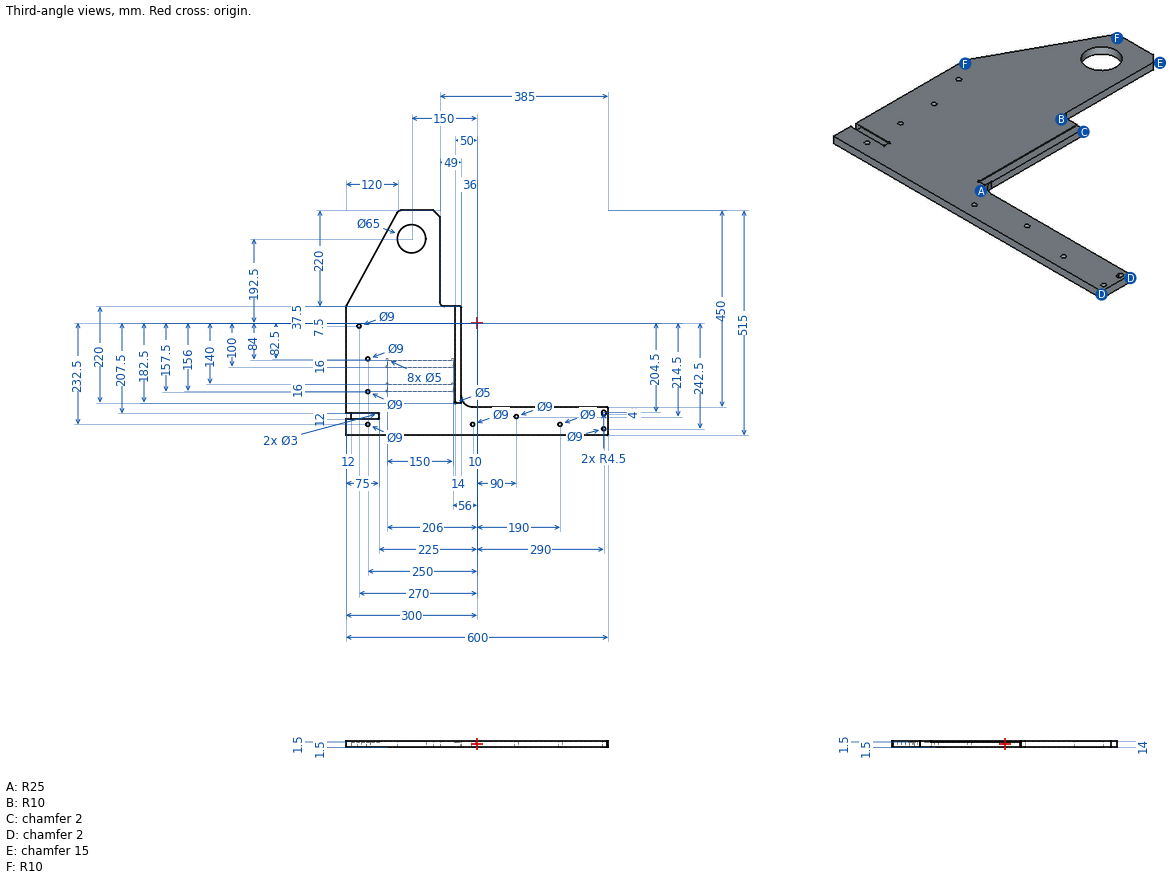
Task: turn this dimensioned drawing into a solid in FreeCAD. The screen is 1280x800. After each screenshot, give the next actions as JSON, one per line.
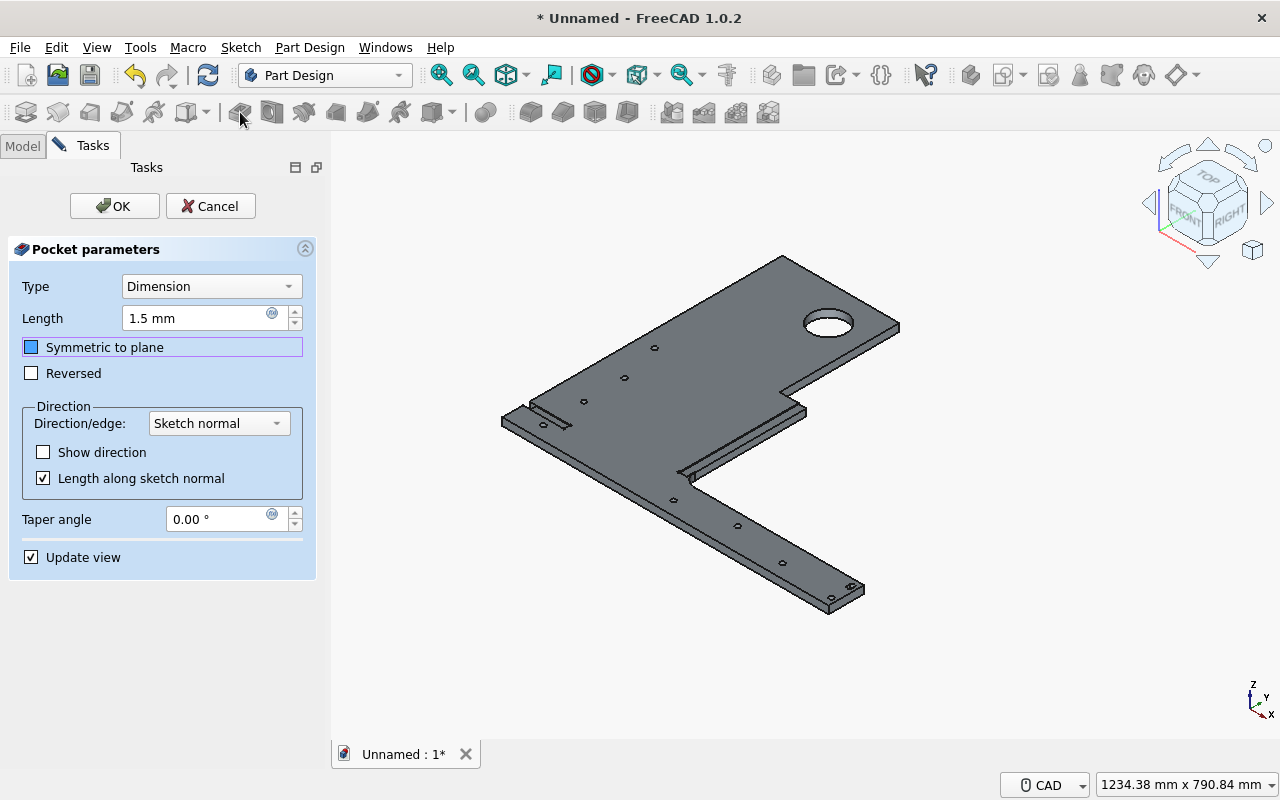
{"action": "left_click", "coordinate": [115, 206]}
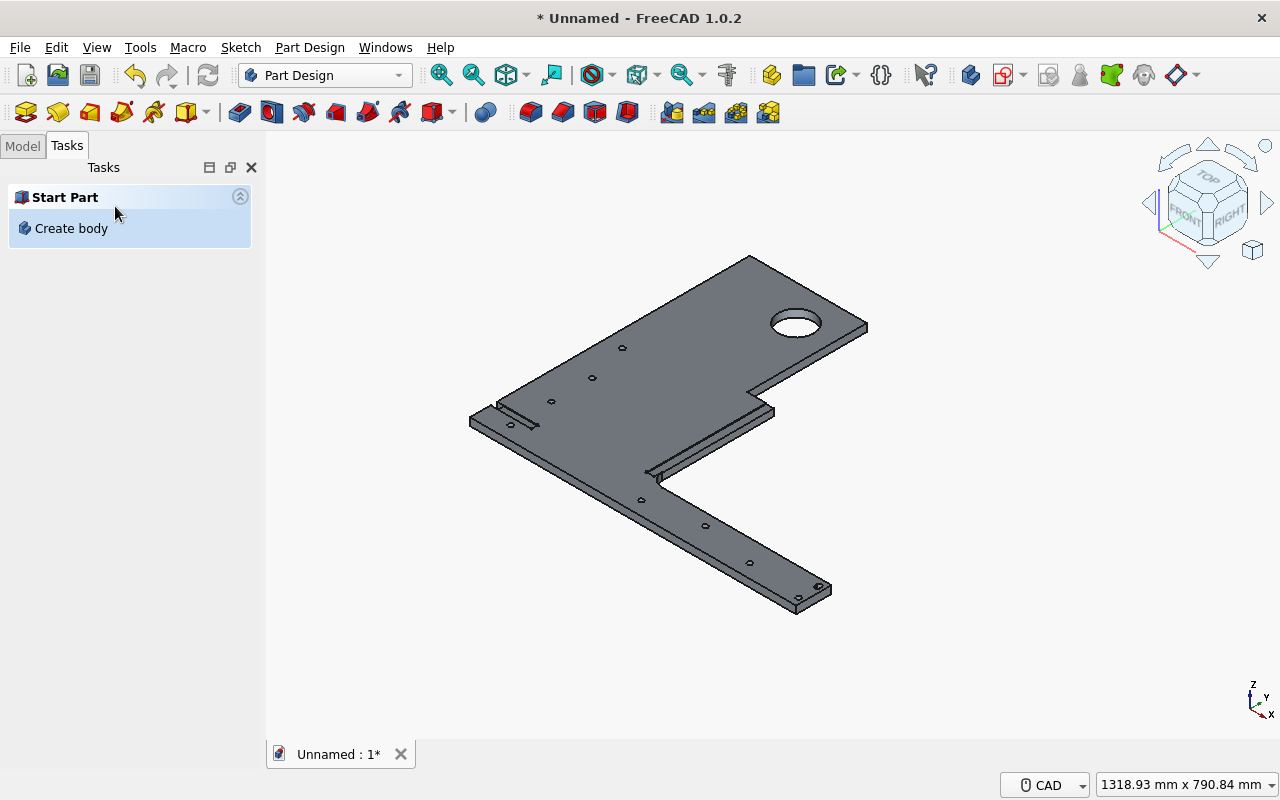
{"action": "scroll", "coordinate": [747, 396], "scroll_direction": "up", "scroll_amount": 7}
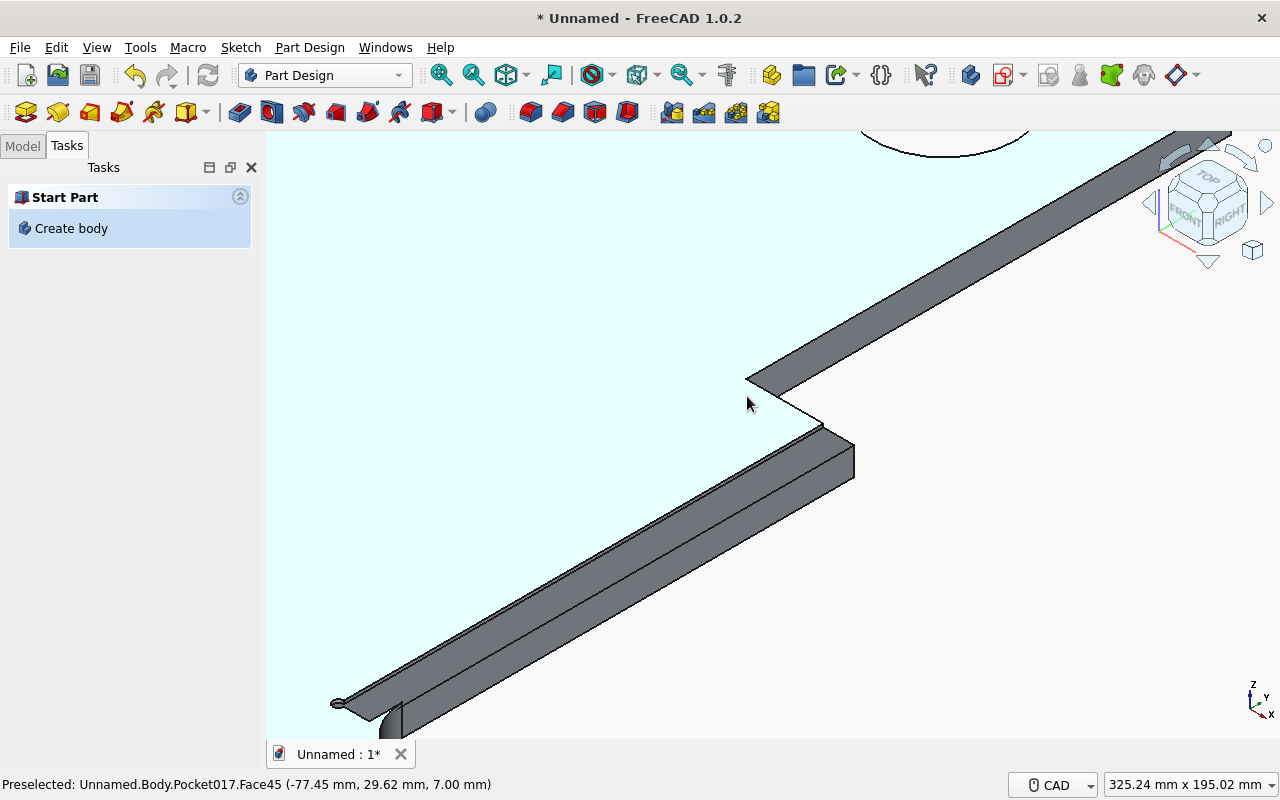
{"action": "left_click", "coordinate": [442, 76]}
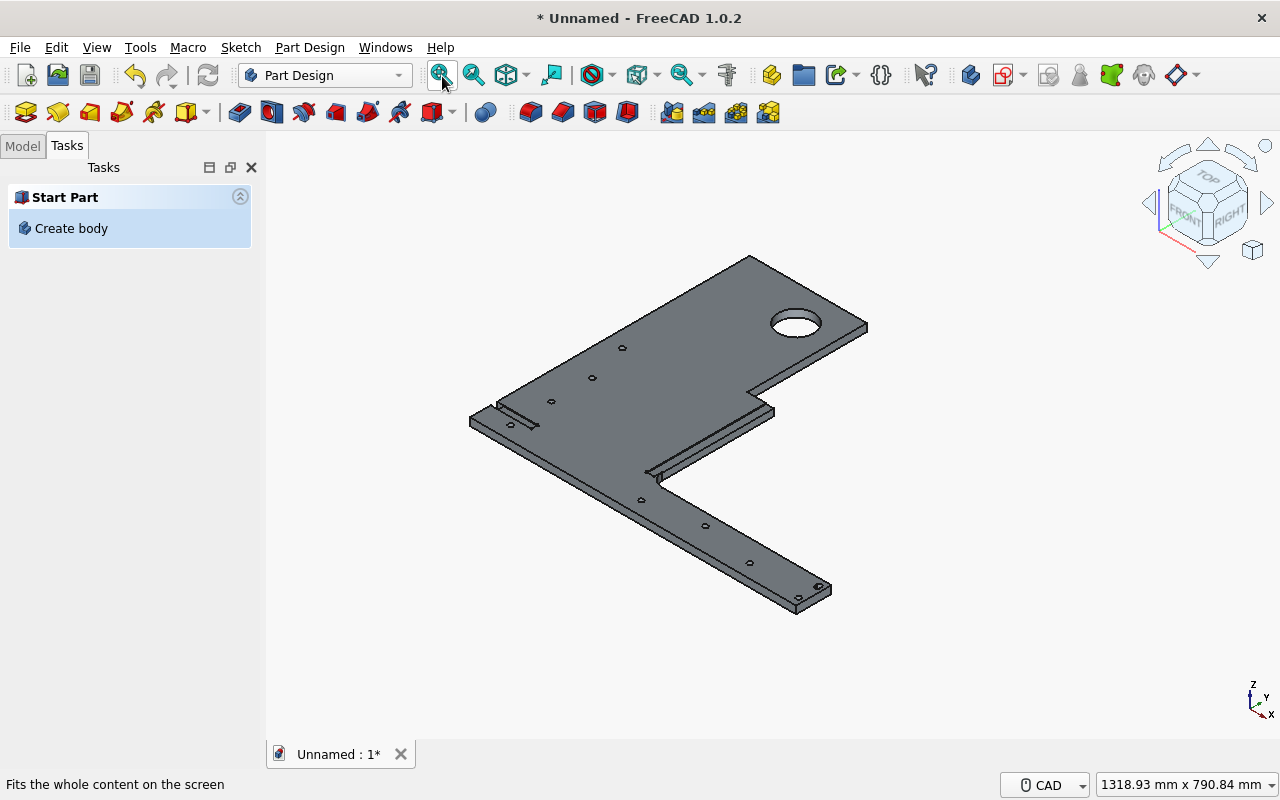
{"action": "key", "text": "2"}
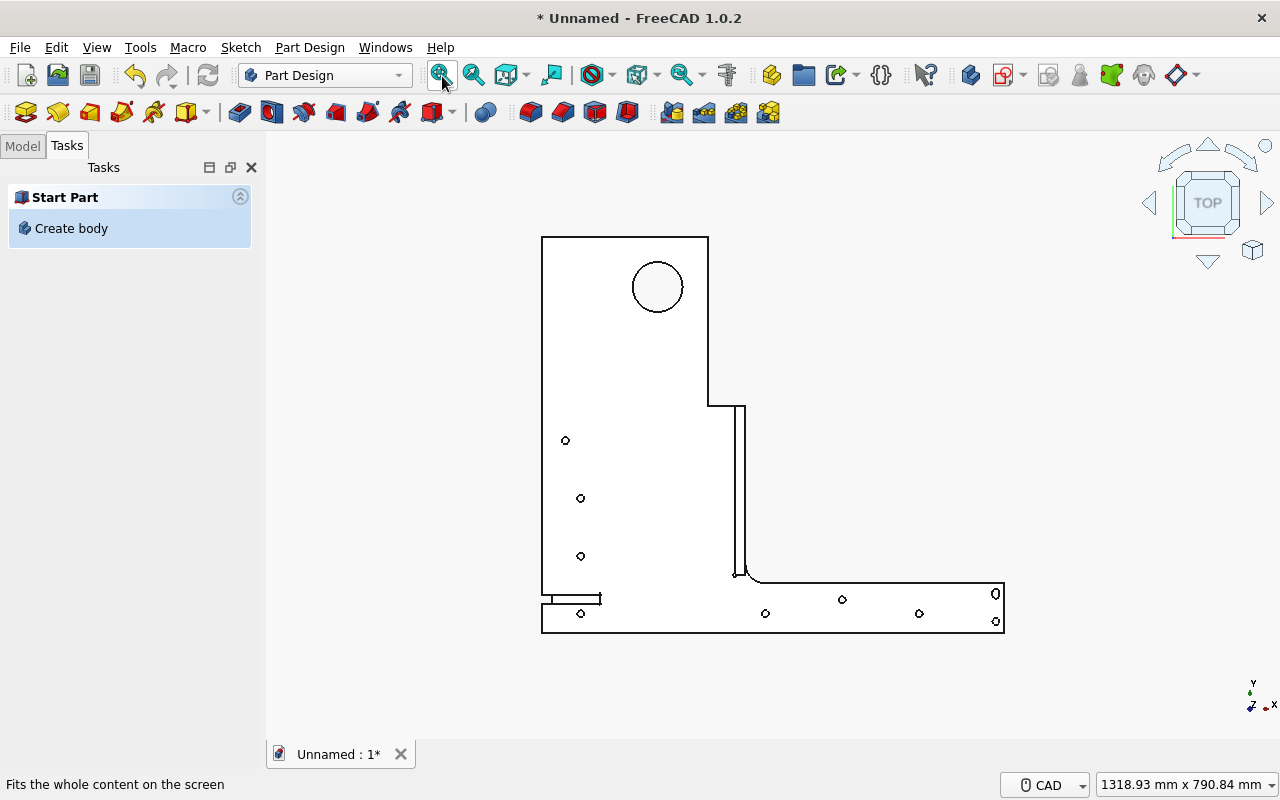
{"action": "scroll", "coordinate": [708, 405], "scroll_direction": "up", "scroll_amount": 7}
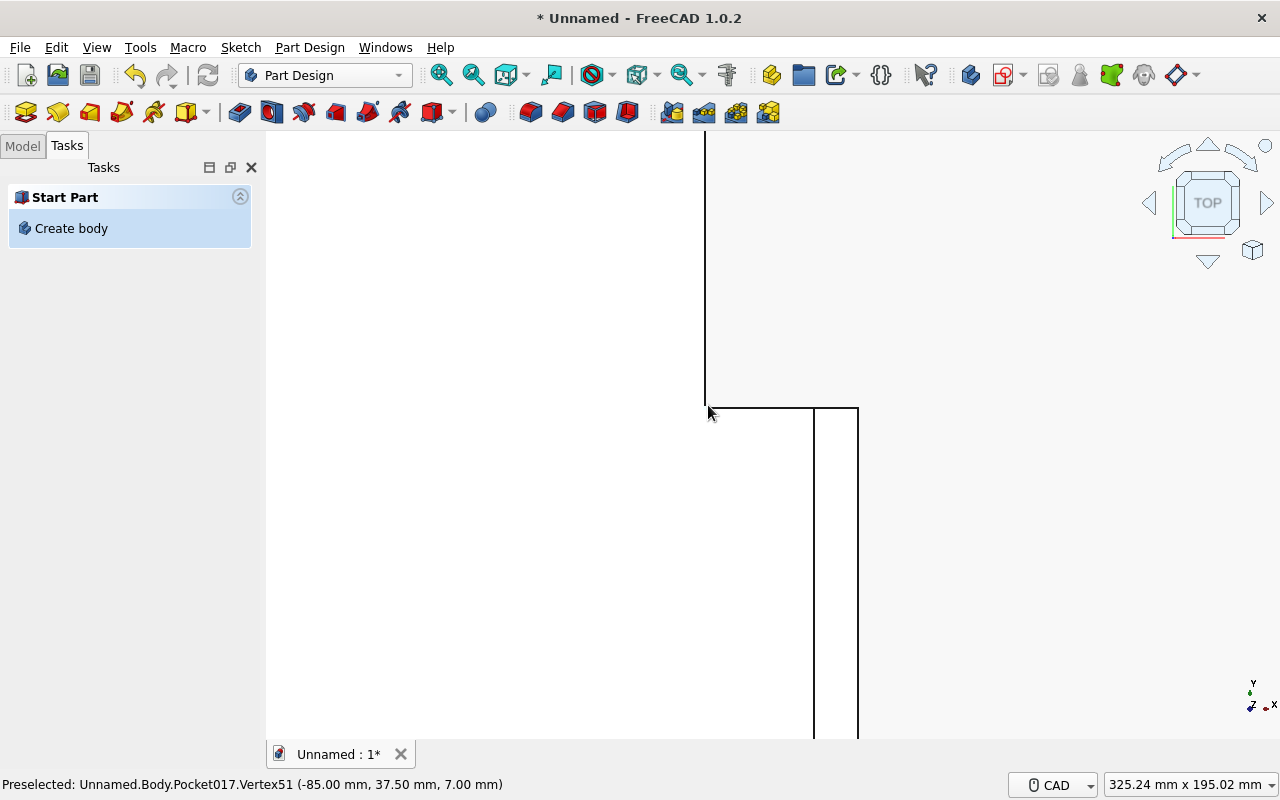
{"action": "left_click", "coordinate": [442, 76]}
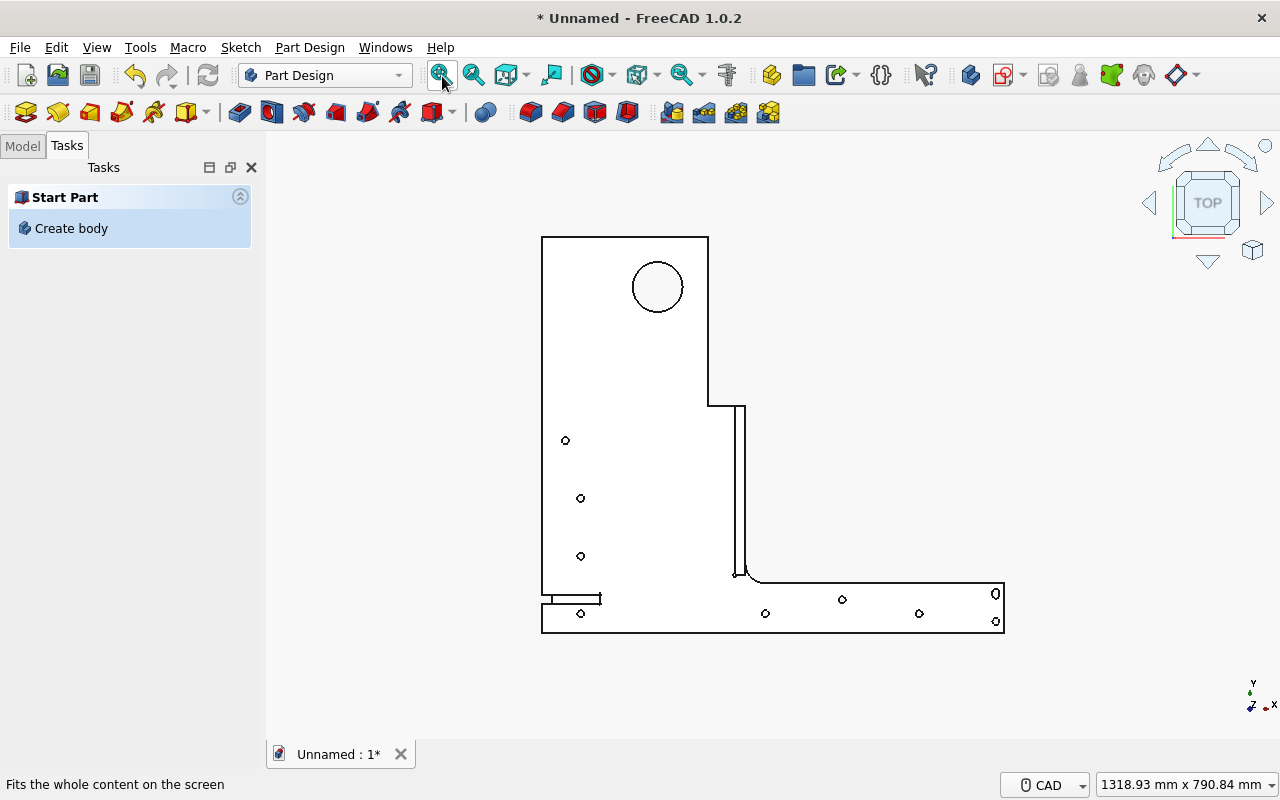
{"action": "key", "text": "0"}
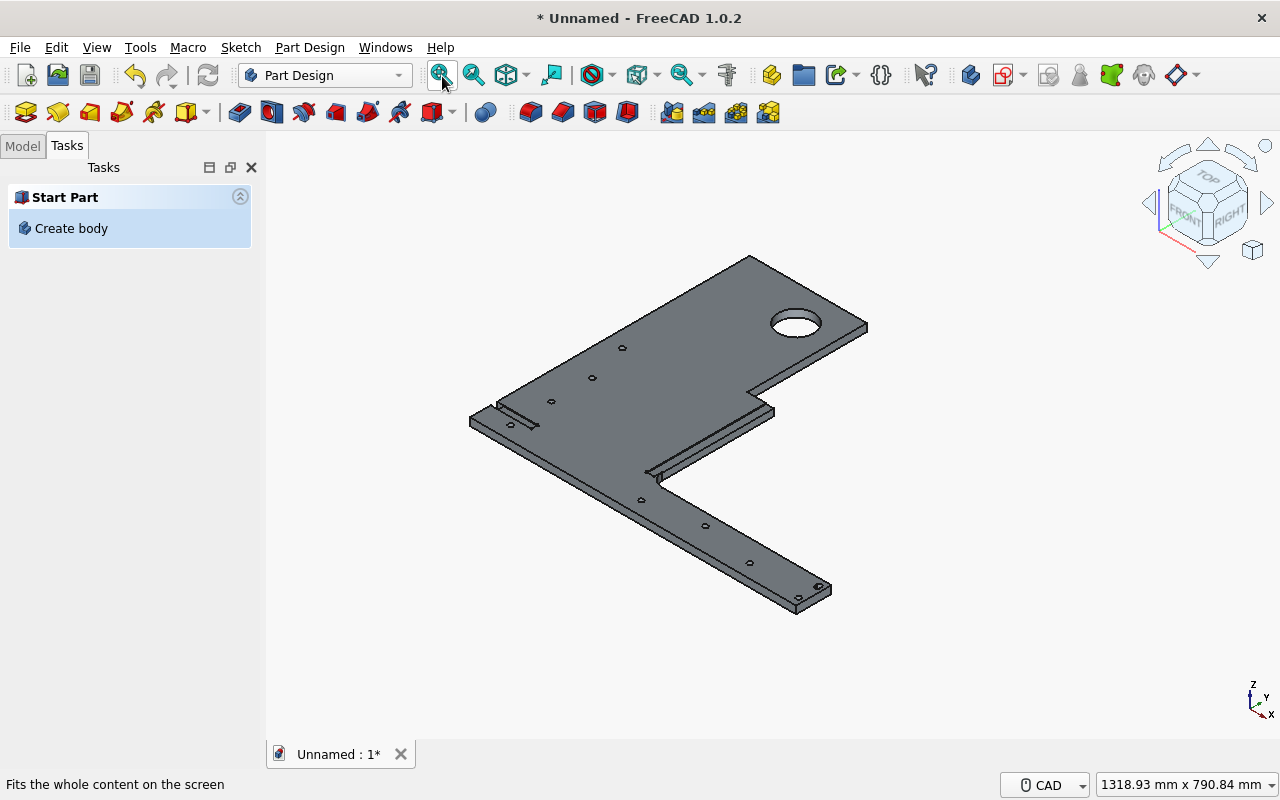
{"action": "scroll", "coordinate": [747, 396], "scroll_direction": "up", "scroll_amount": 7}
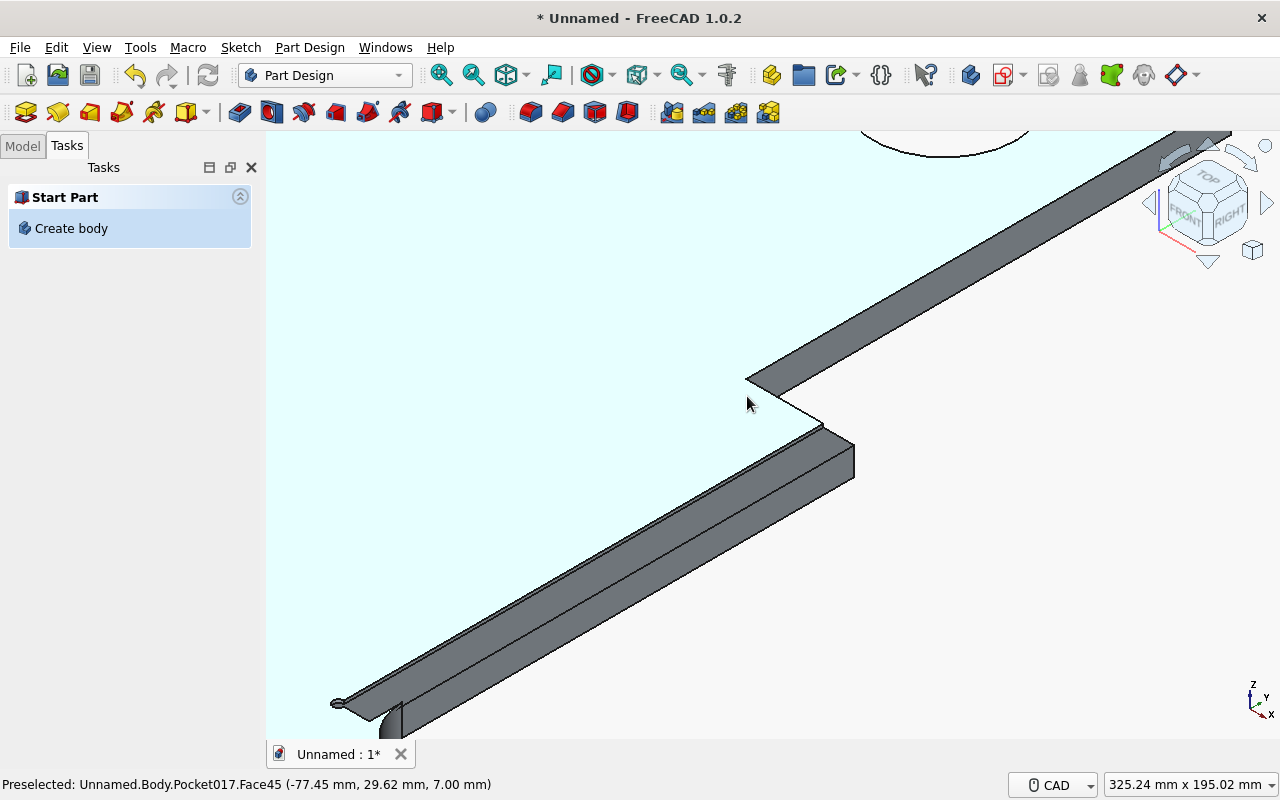
{"action": "left_click", "coordinate": [442, 76]}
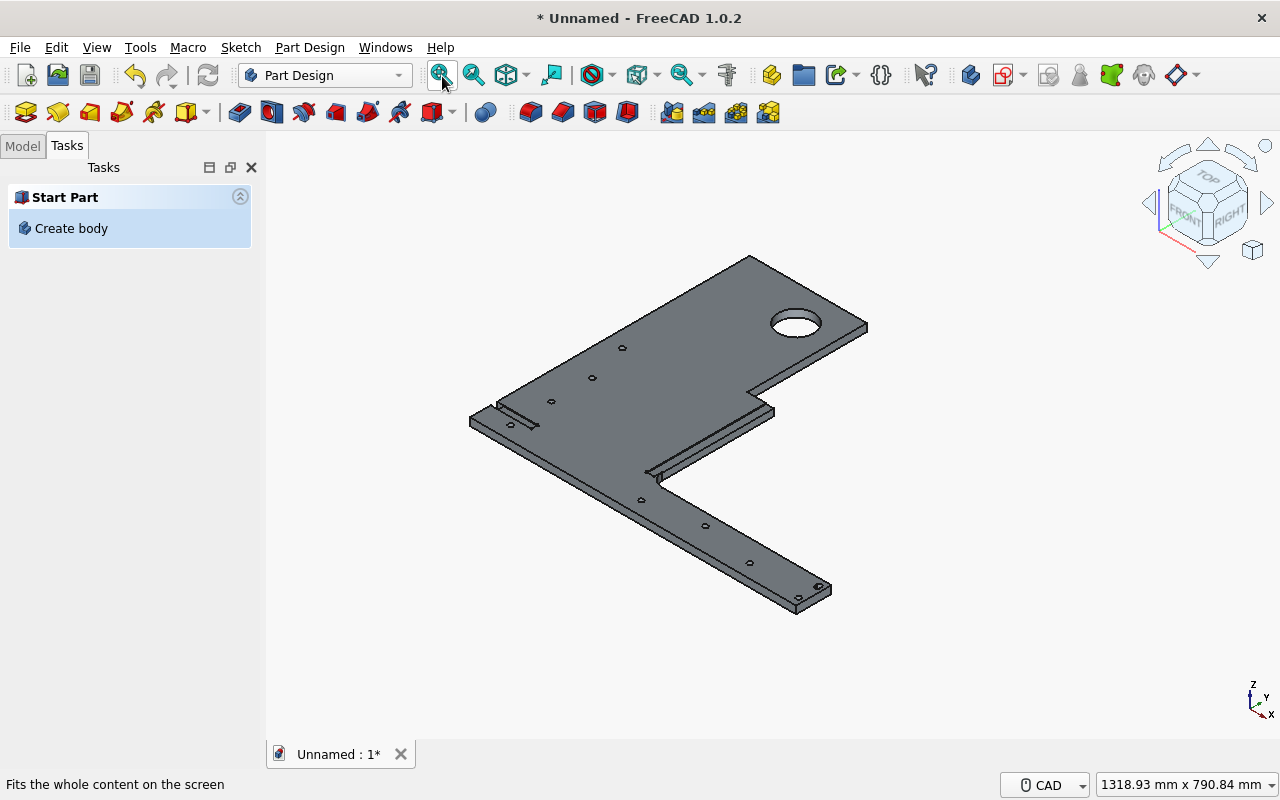
{"action": "key", "text": "1"}